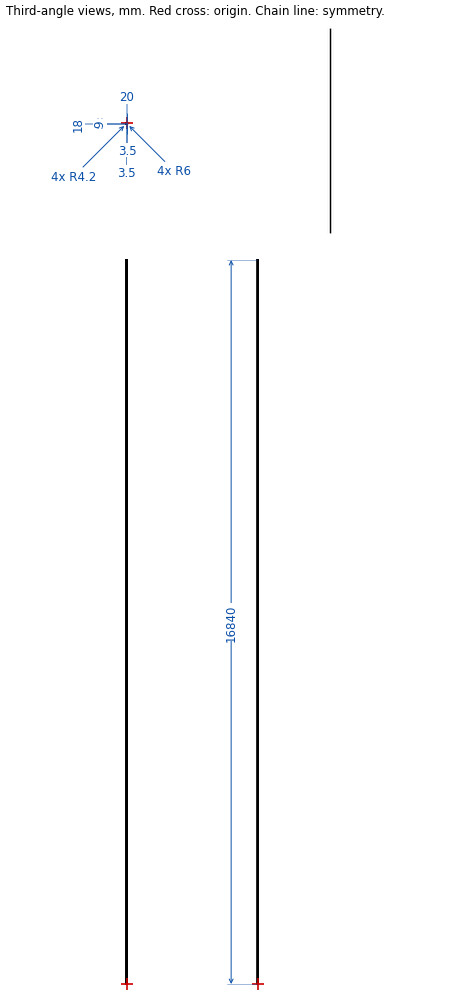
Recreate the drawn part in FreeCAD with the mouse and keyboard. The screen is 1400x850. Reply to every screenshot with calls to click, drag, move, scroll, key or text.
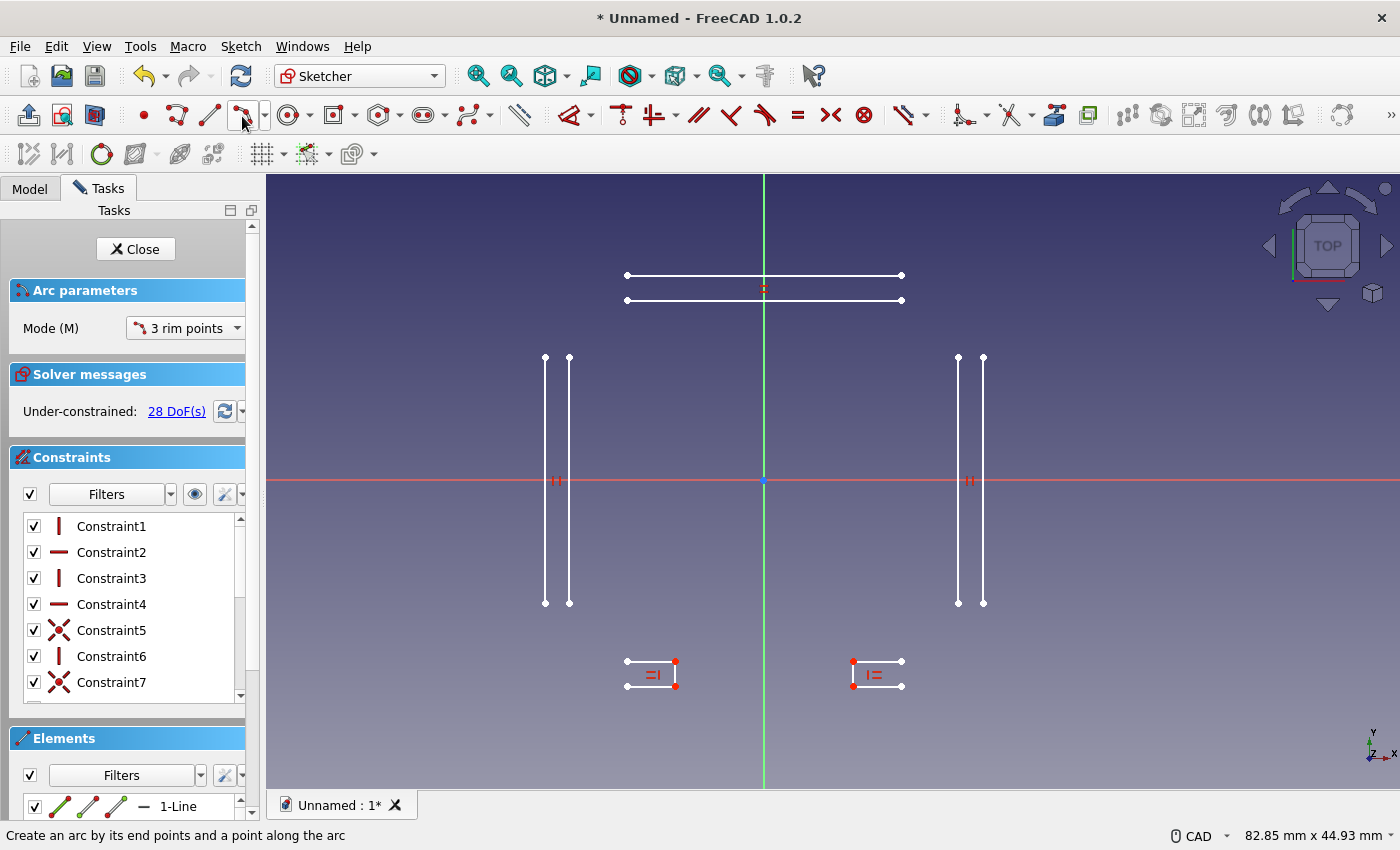
click(569, 358)
click(627, 301)
click(586, 316)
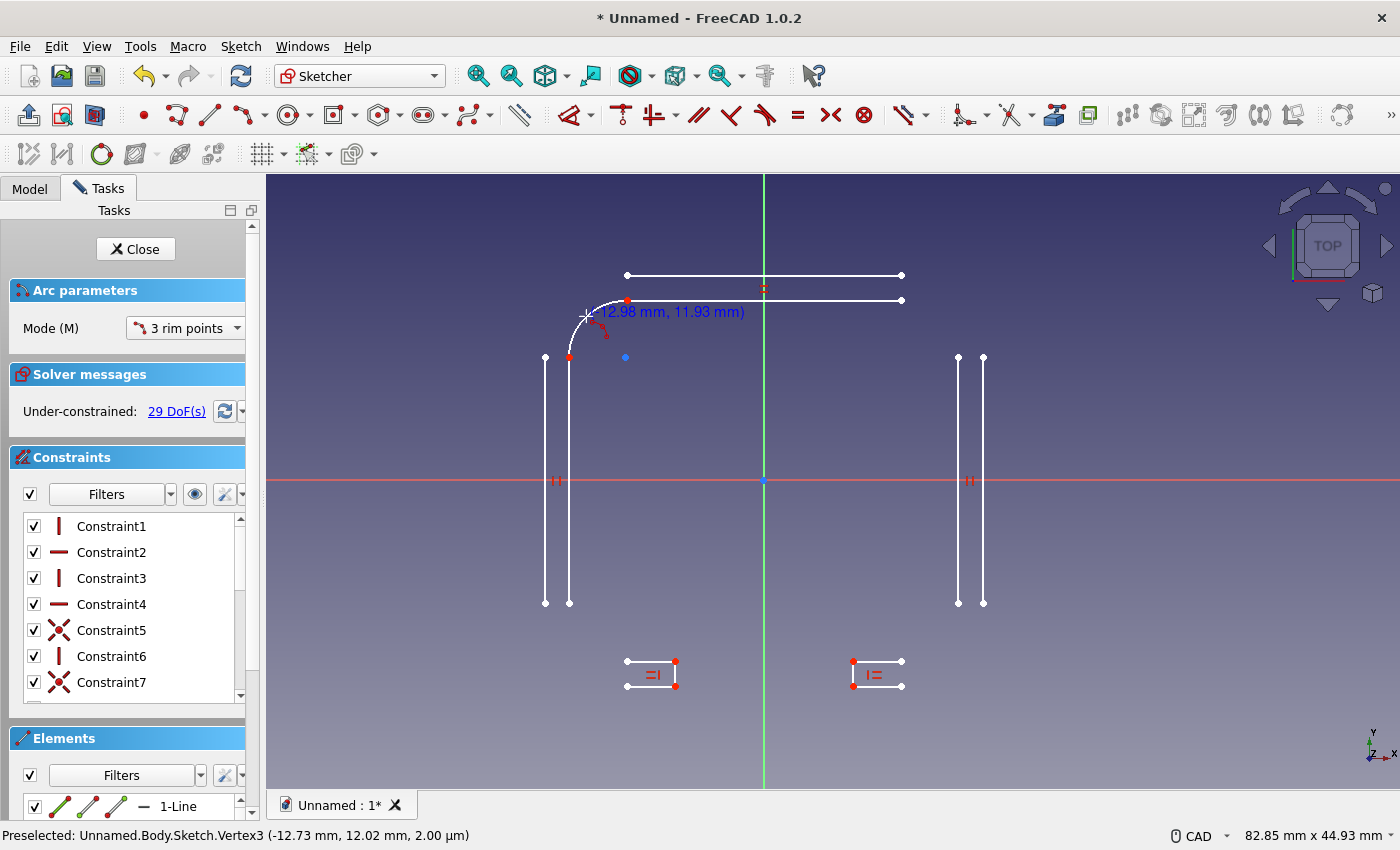
click(901, 301)
click(958, 358)
click(941, 316)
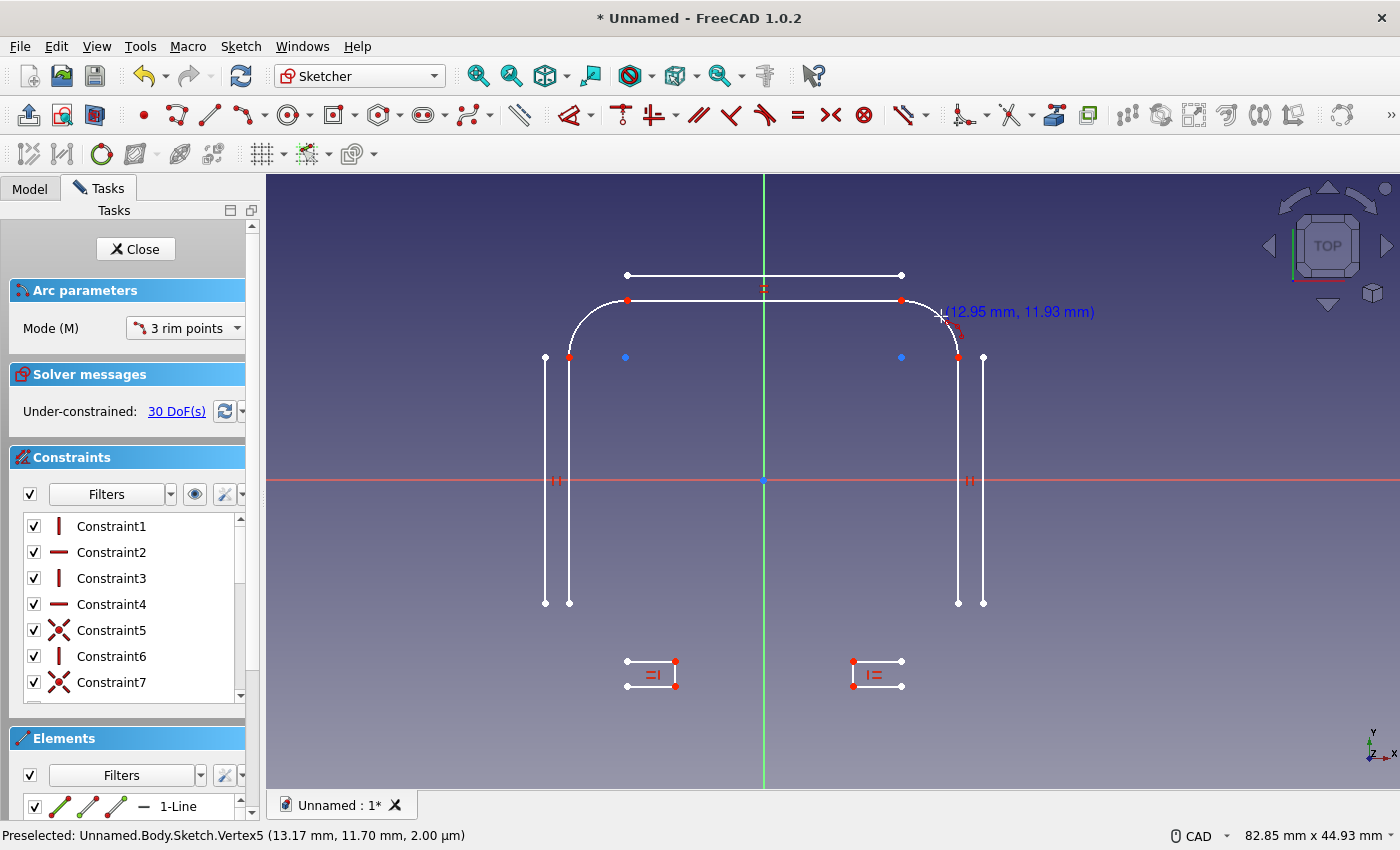
click(958, 604)
click(901, 662)
click(941, 644)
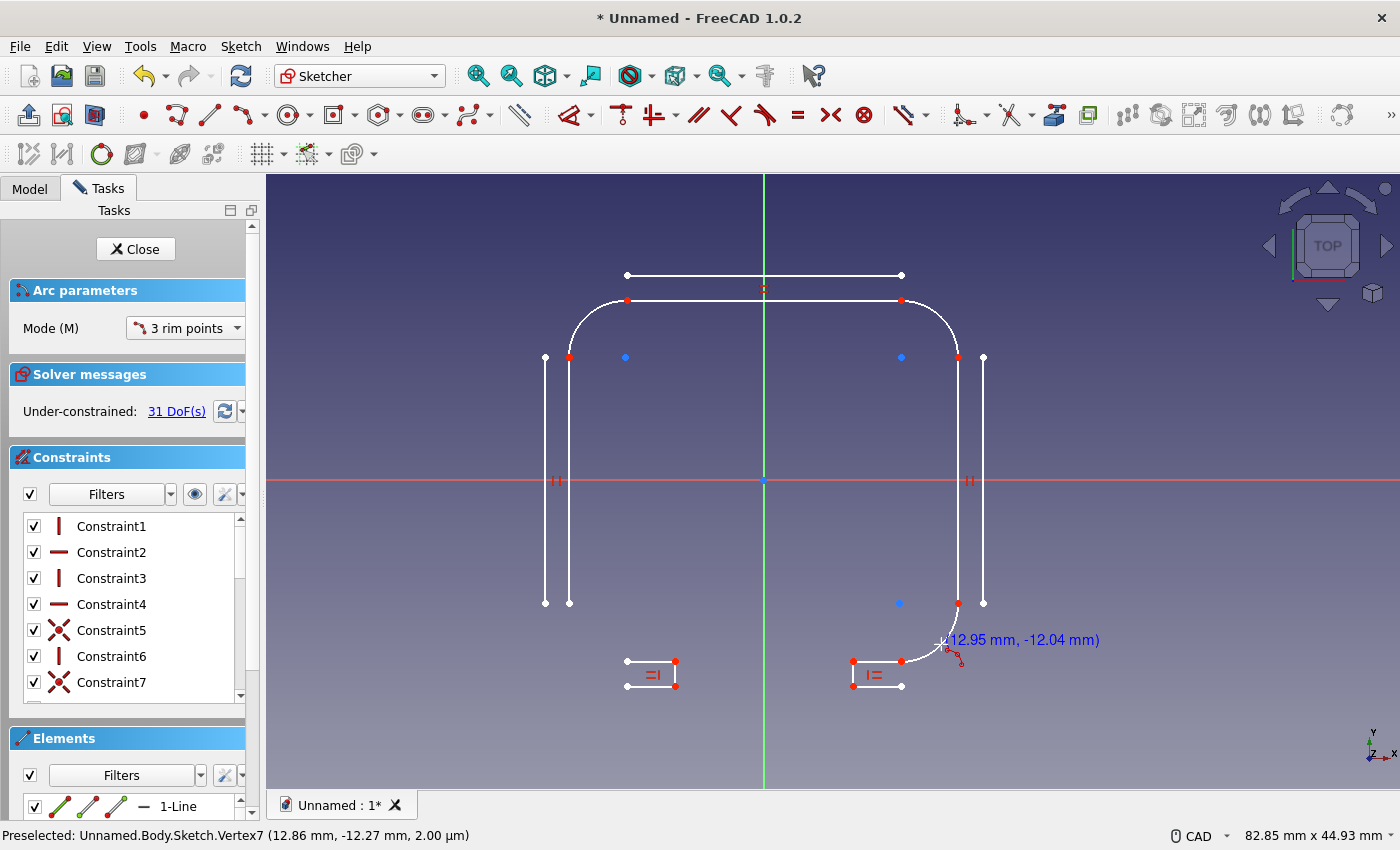
click(901, 687)
click(983, 604)
click(959, 662)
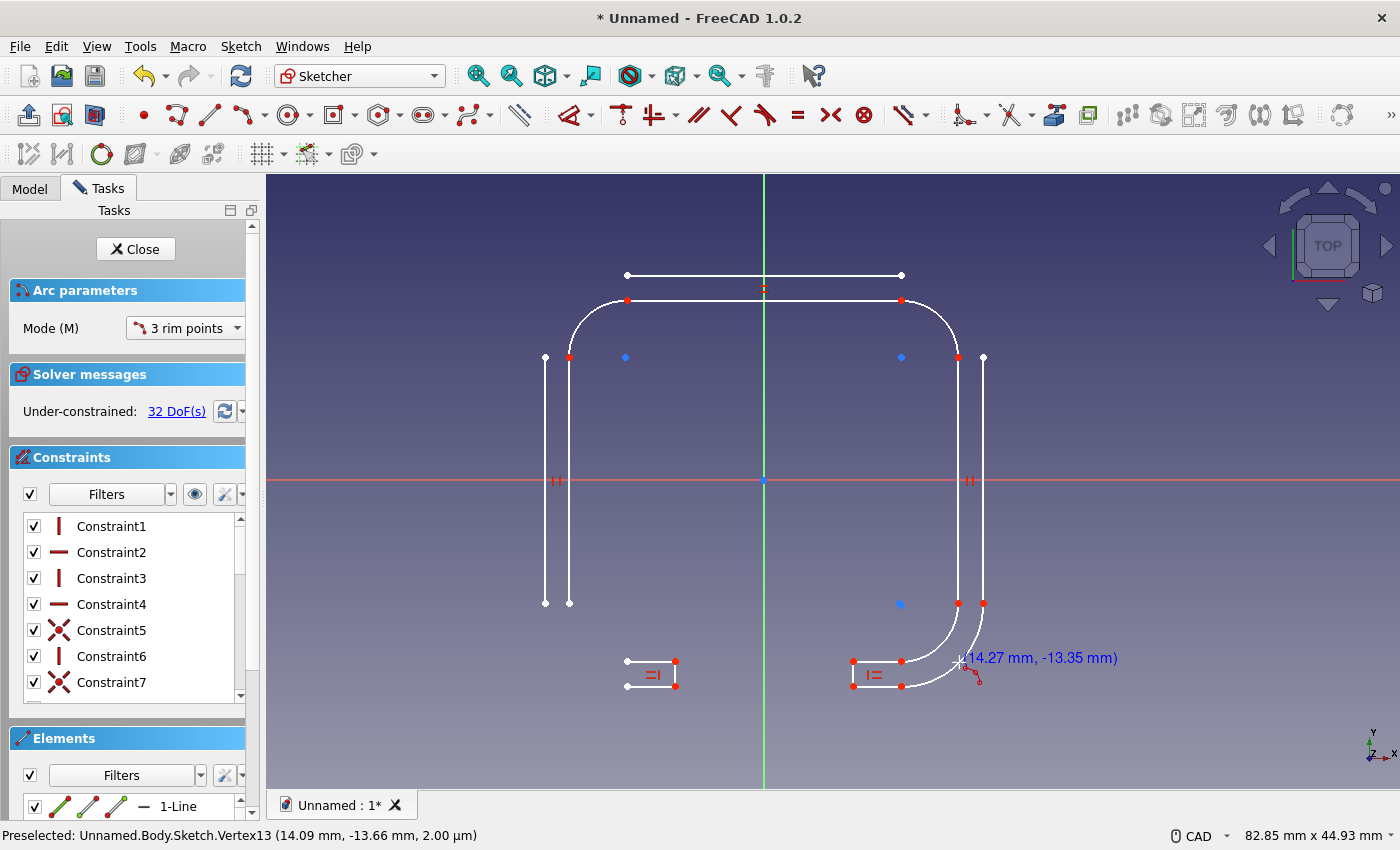
click(983, 358)
click(901, 276)
click(959, 299)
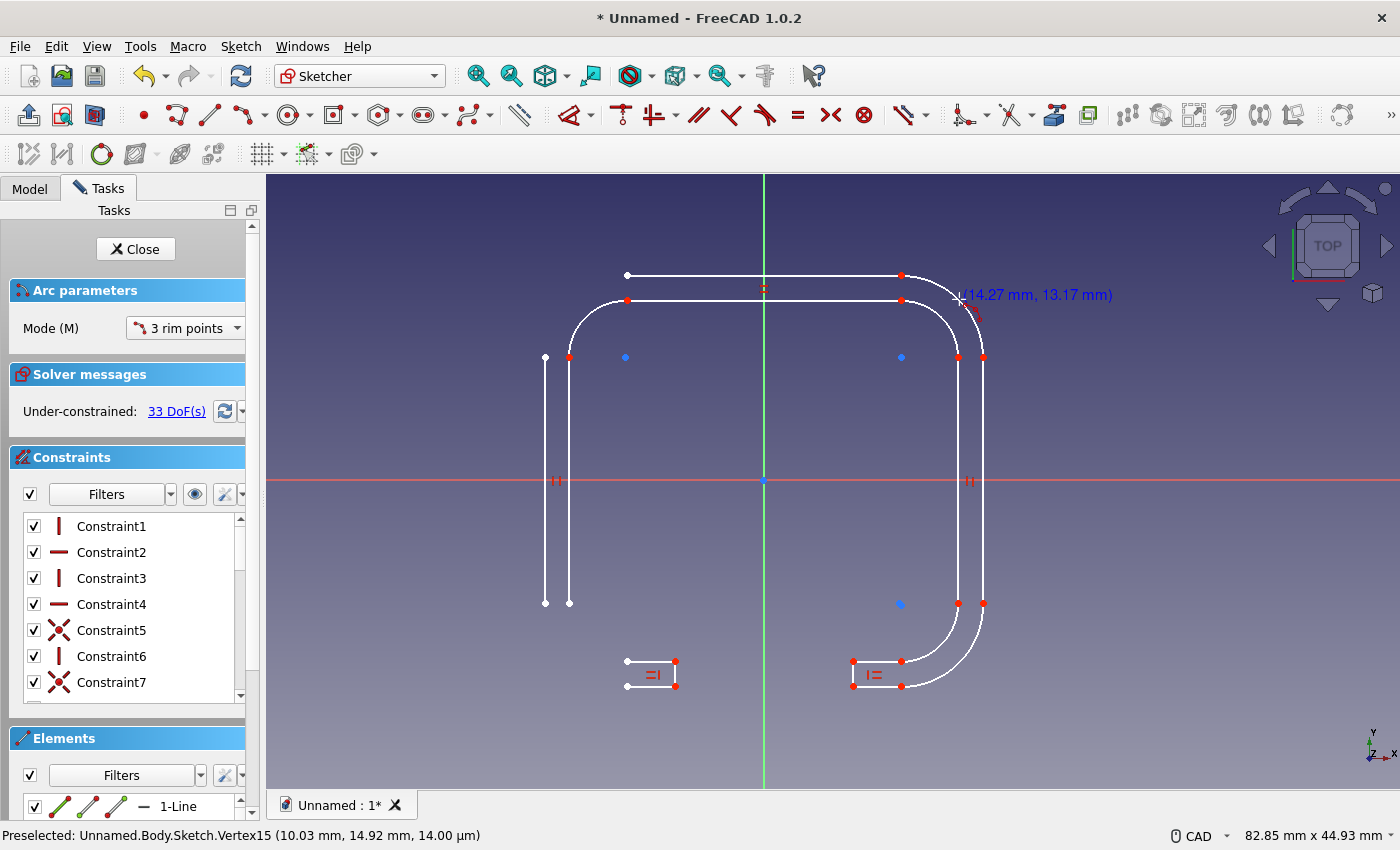
click(627, 276)
click(545, 358)
click(569, 299)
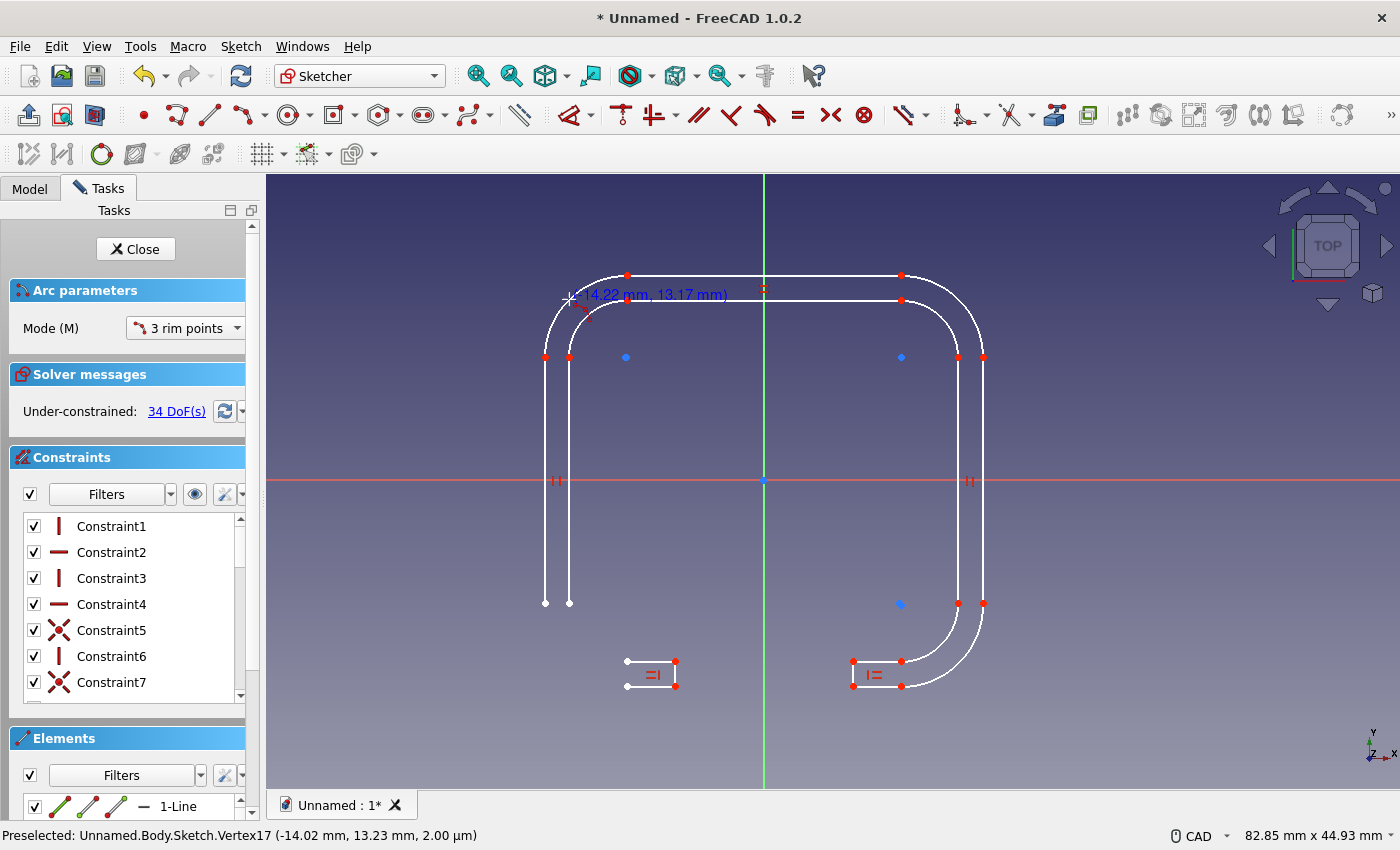
click(545, 604)
click(627, 687)
click(569, 662)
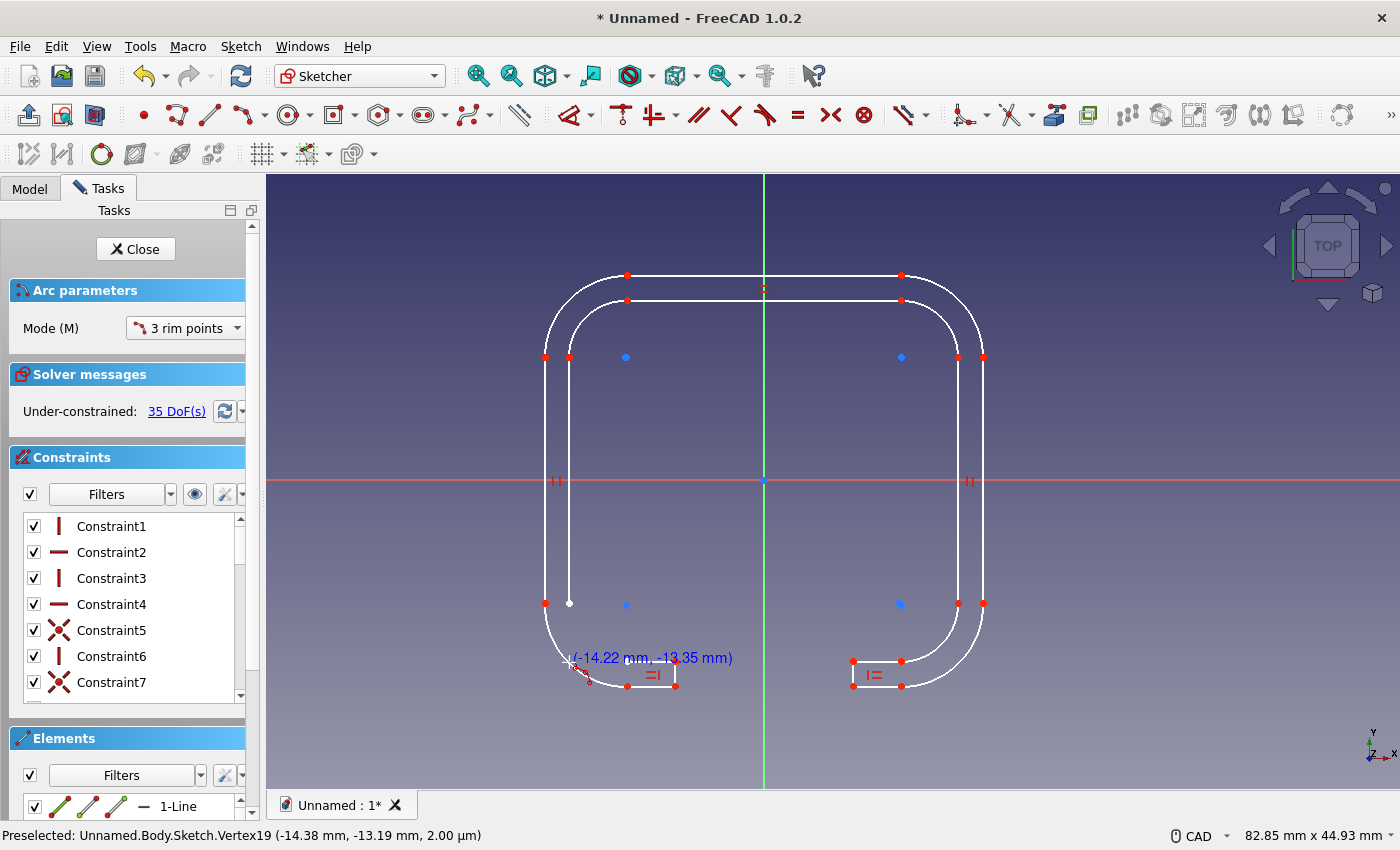
click(627, 662)
click(569, 604)
click(586, 644)
key(Escape)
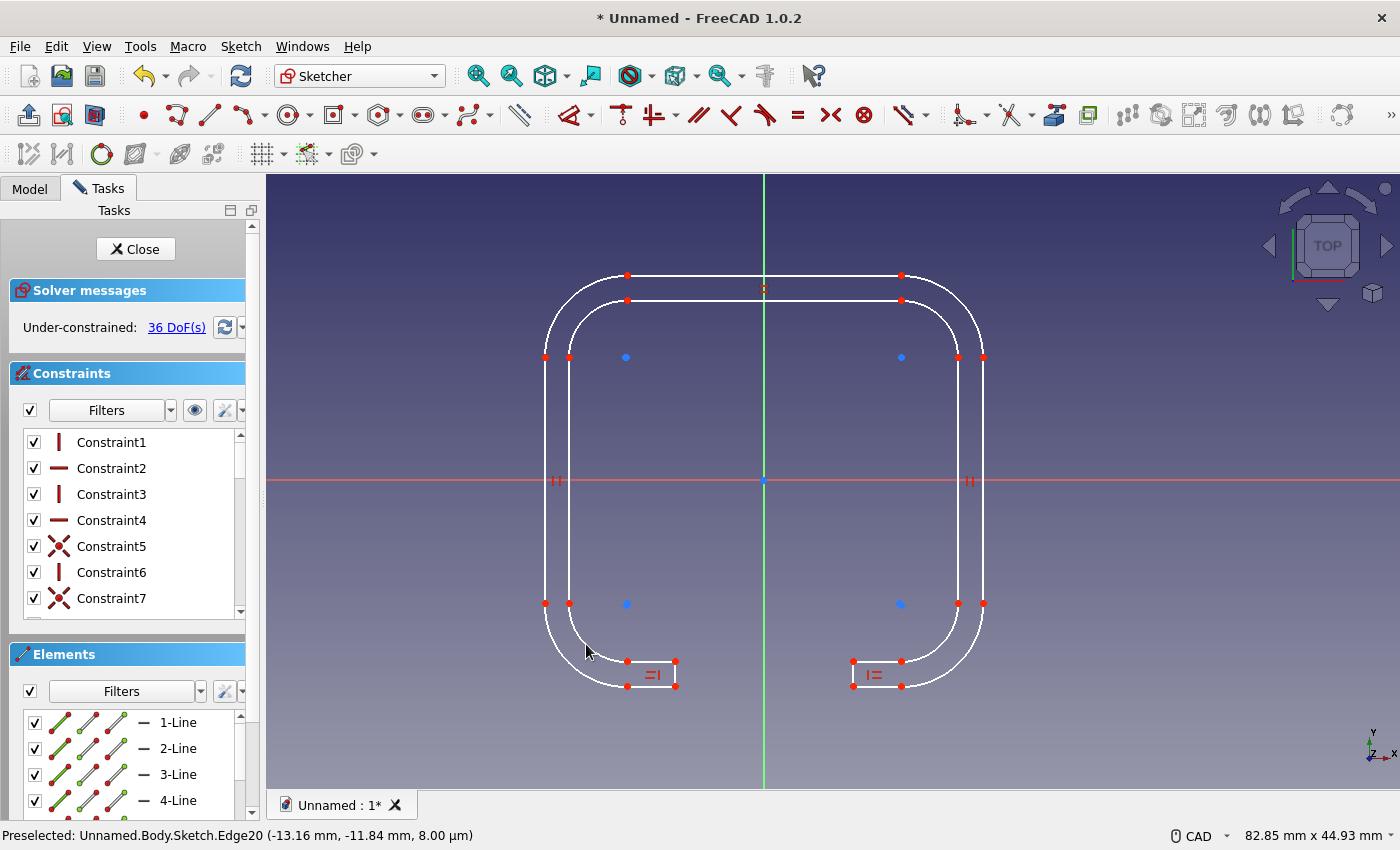
click(569, 530)